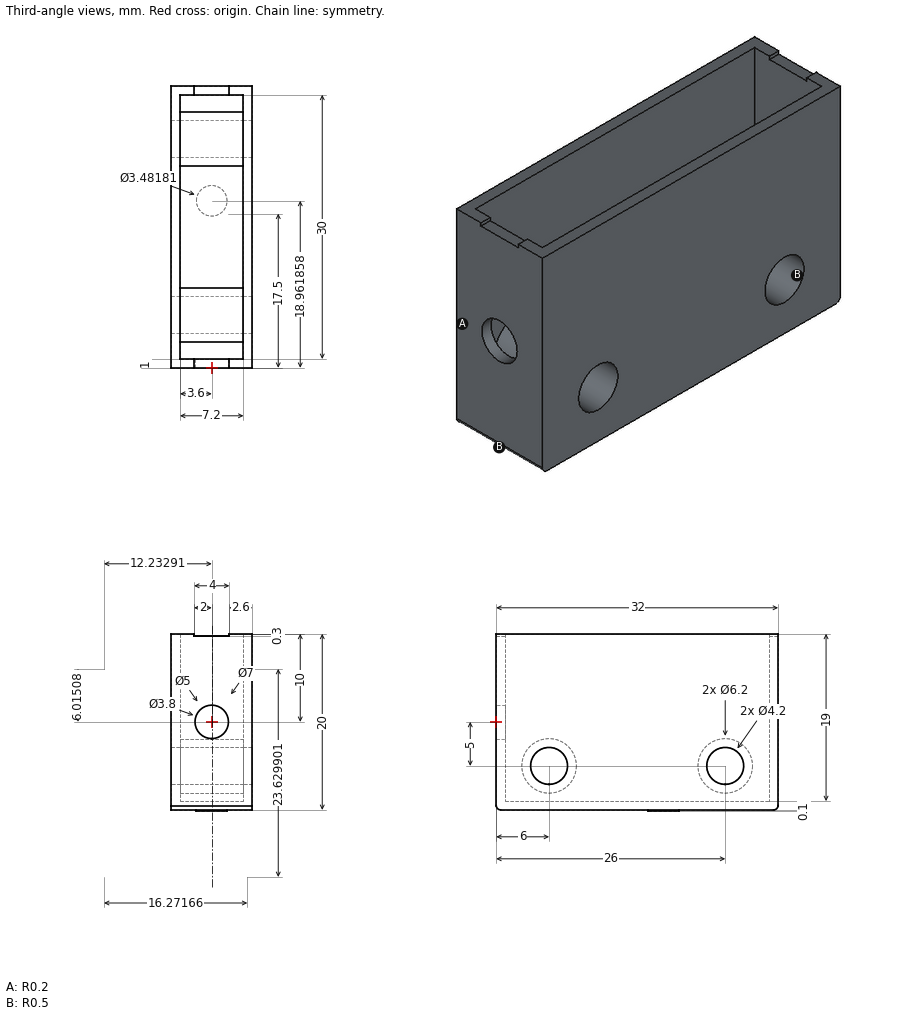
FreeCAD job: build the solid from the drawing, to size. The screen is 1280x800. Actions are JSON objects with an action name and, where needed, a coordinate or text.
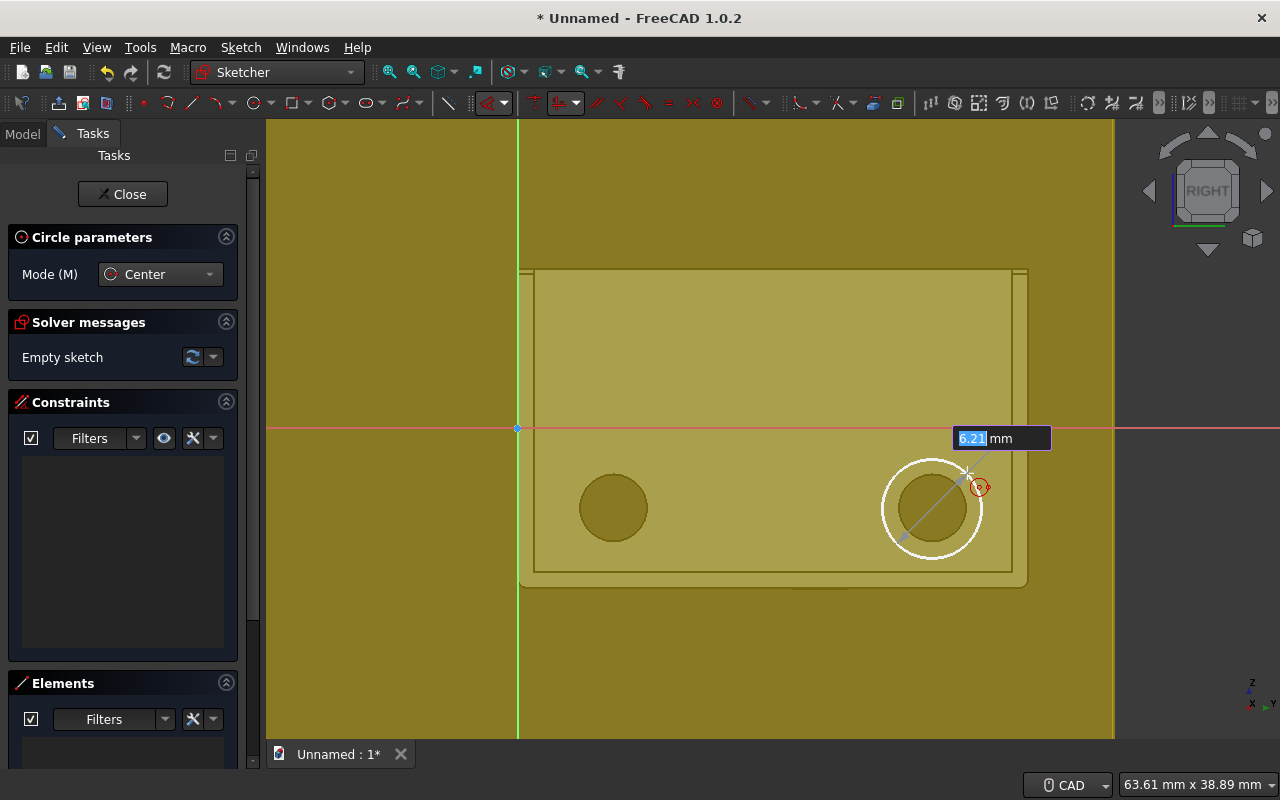
{"action": "type", "text": "6.2"}
{"action": "key", "text": "Return"}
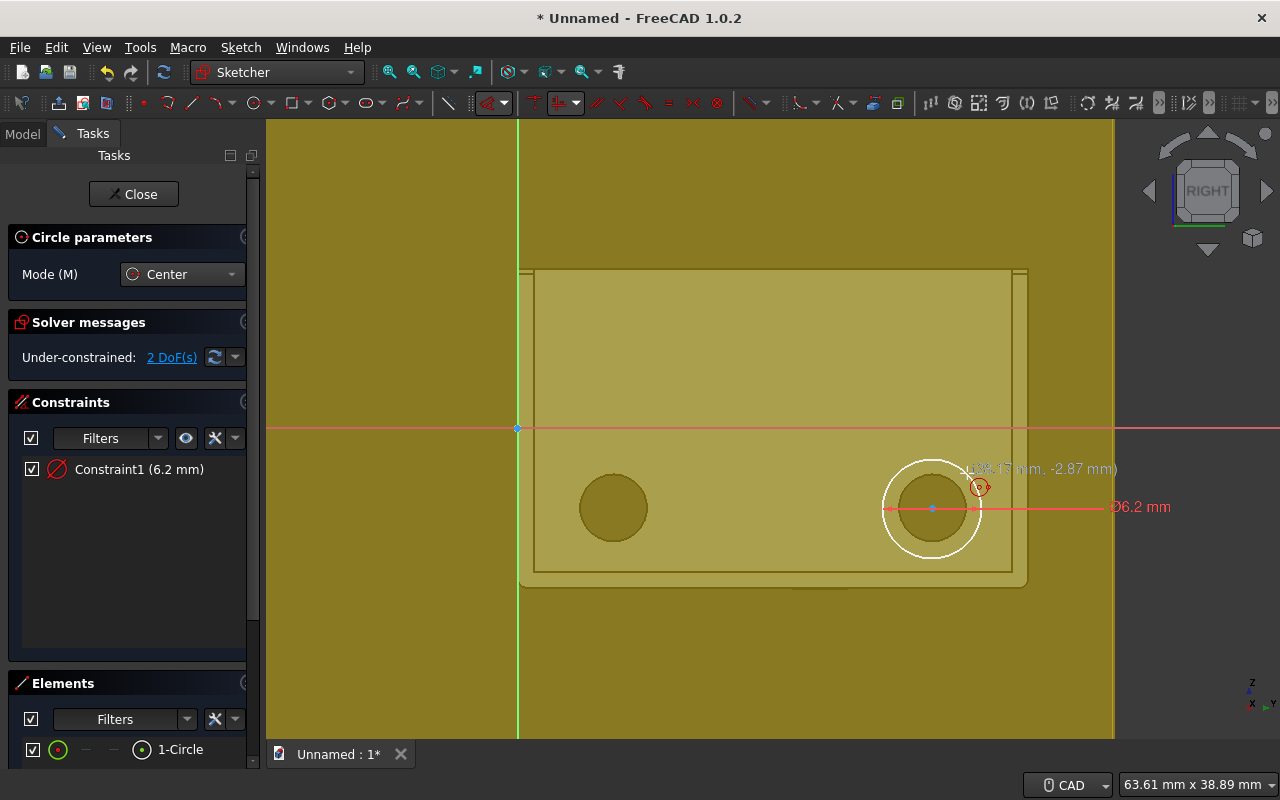
{"action": "left_click", "coordinate": [614, 508]}
{"action": "mouse_move", "coordinate": [649, 473]}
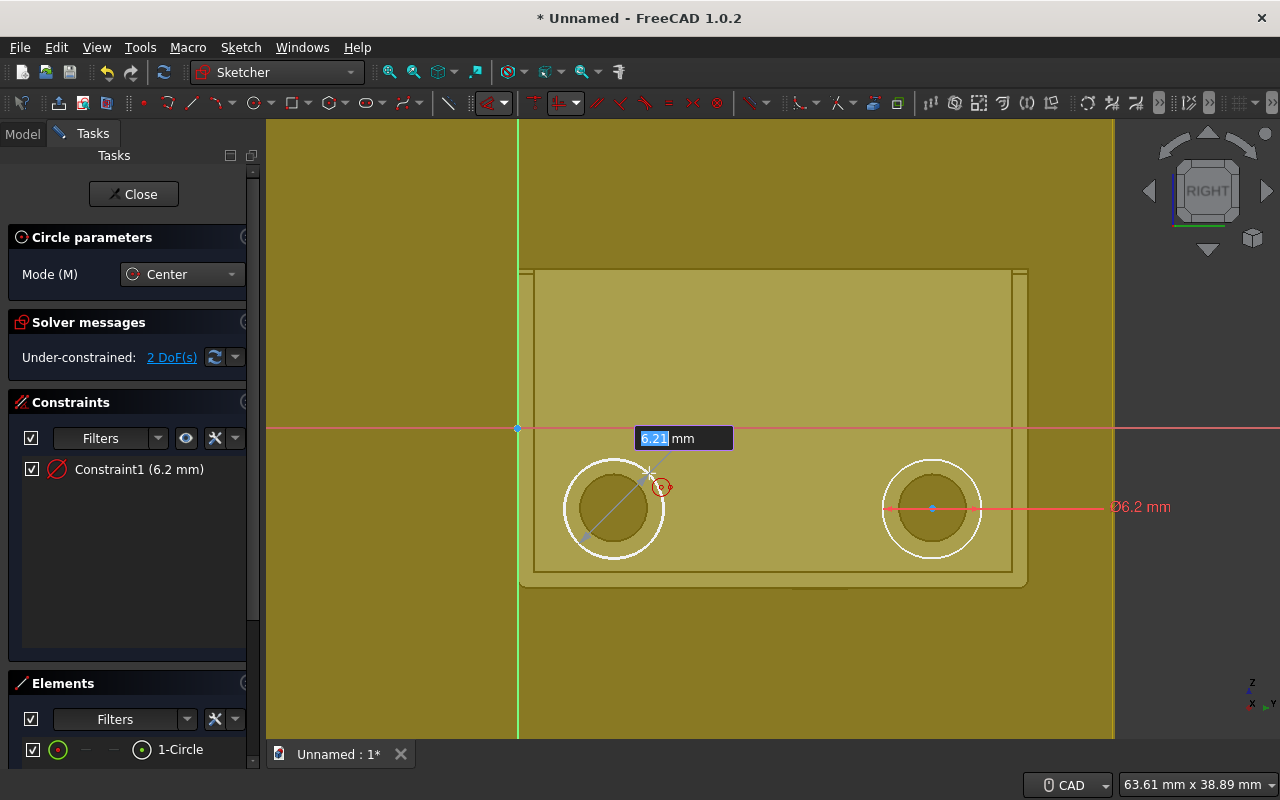
{"action": "type", "text": "6.2"}
{"action": "key", "text": "Return"}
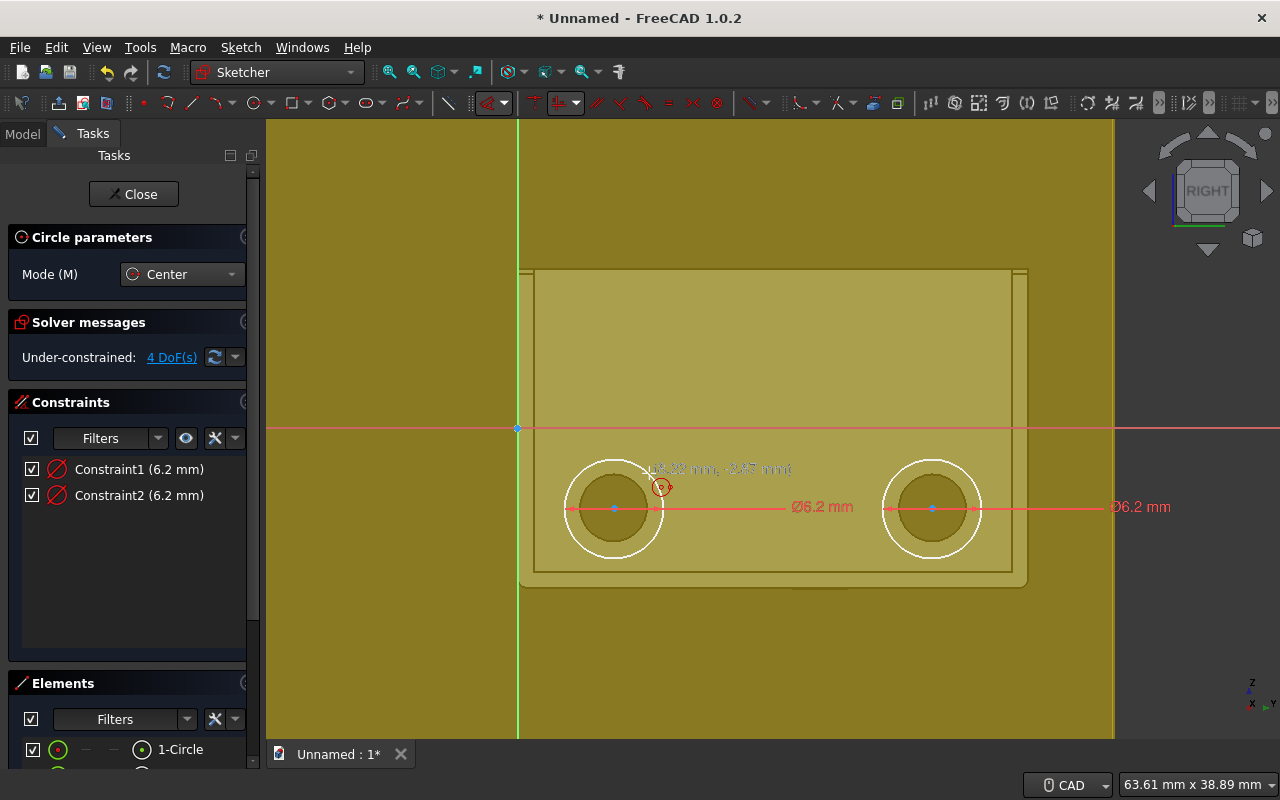
{"action": "left_click", "coordinate": [932, 509]}
{"action": "mouse_move", "coordinate": [956, 484]}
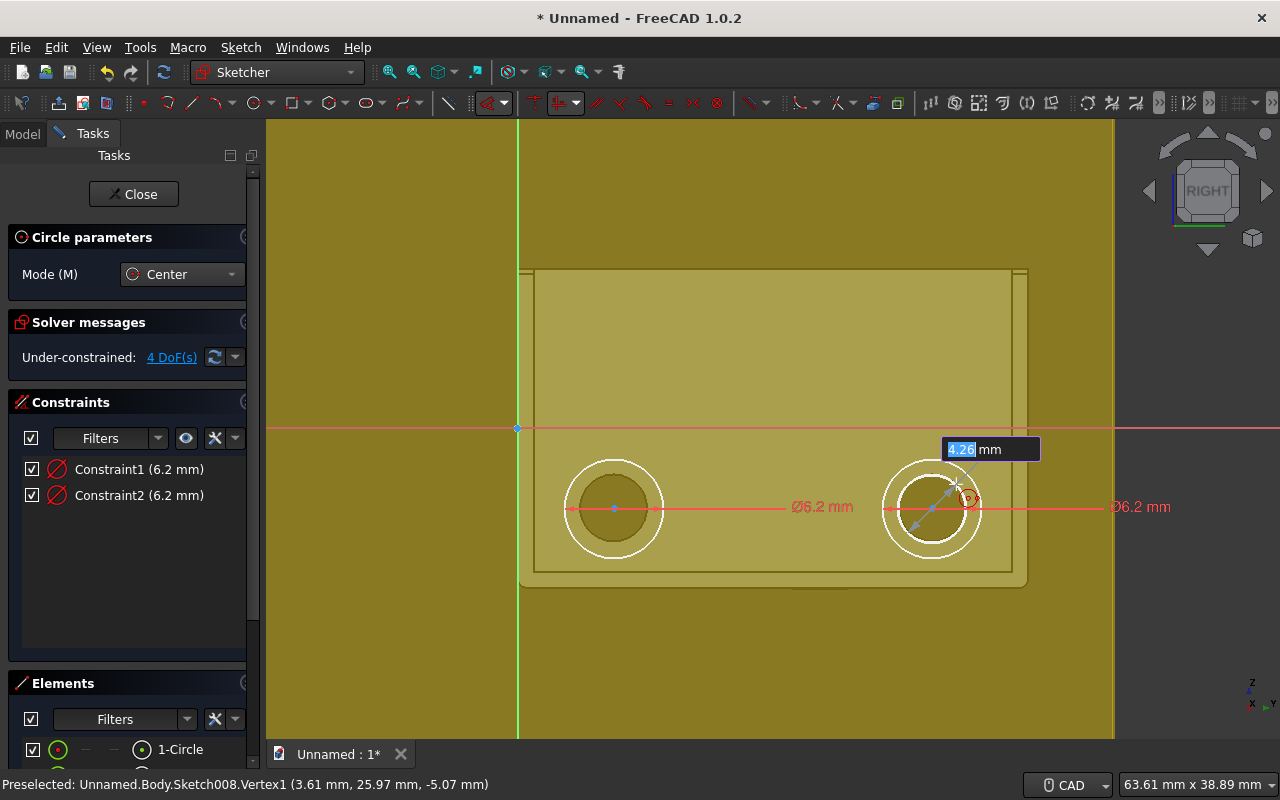
{"action": "type", "text": "4.2"}
{"action": "key", "text": "Return"}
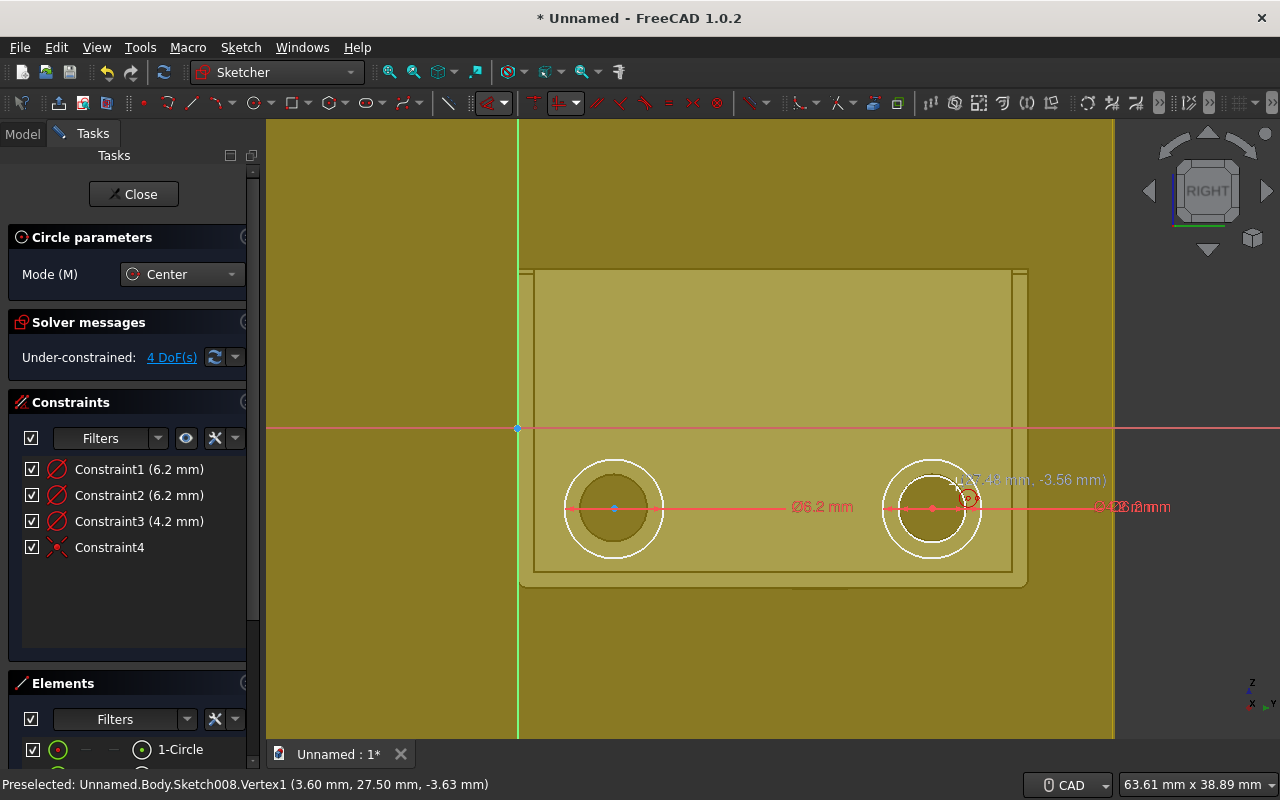
{"action": "left_click", "coordinate": [614, 509]}
{"action": "mouse_move", "coordinate": [637, 484]}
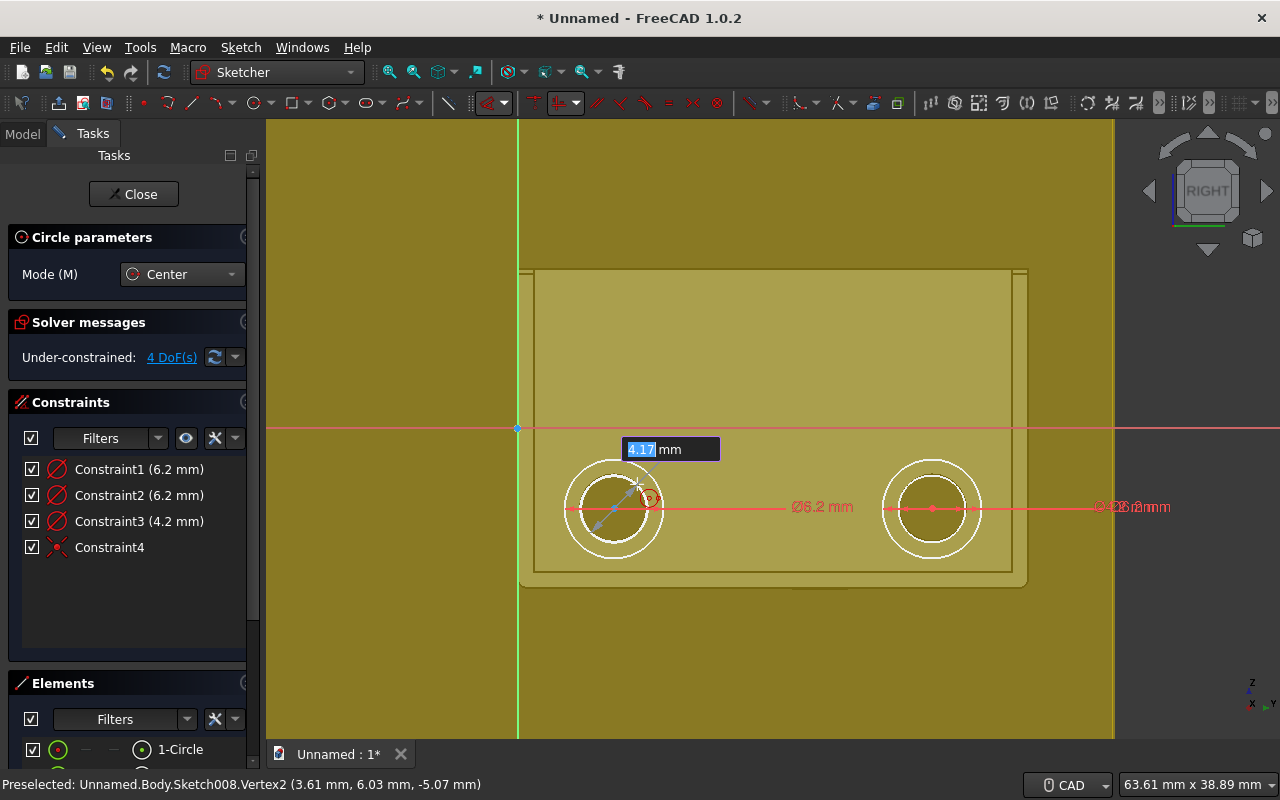
{"action": "type", "text": "4.2"}
{"action": "key", "text": "Return"}
{"action": "key", "text": "Escape"}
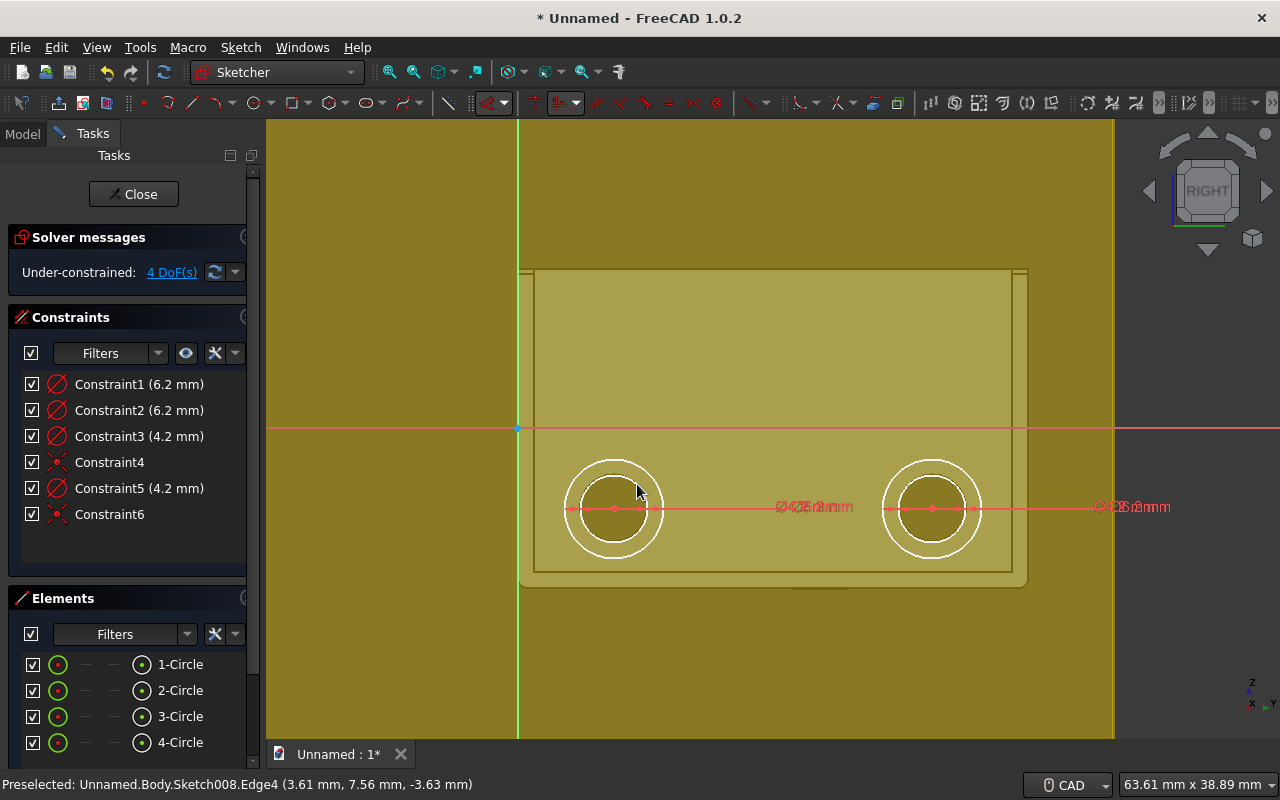
{"action": "left_click", "coordinate": [932, 509]}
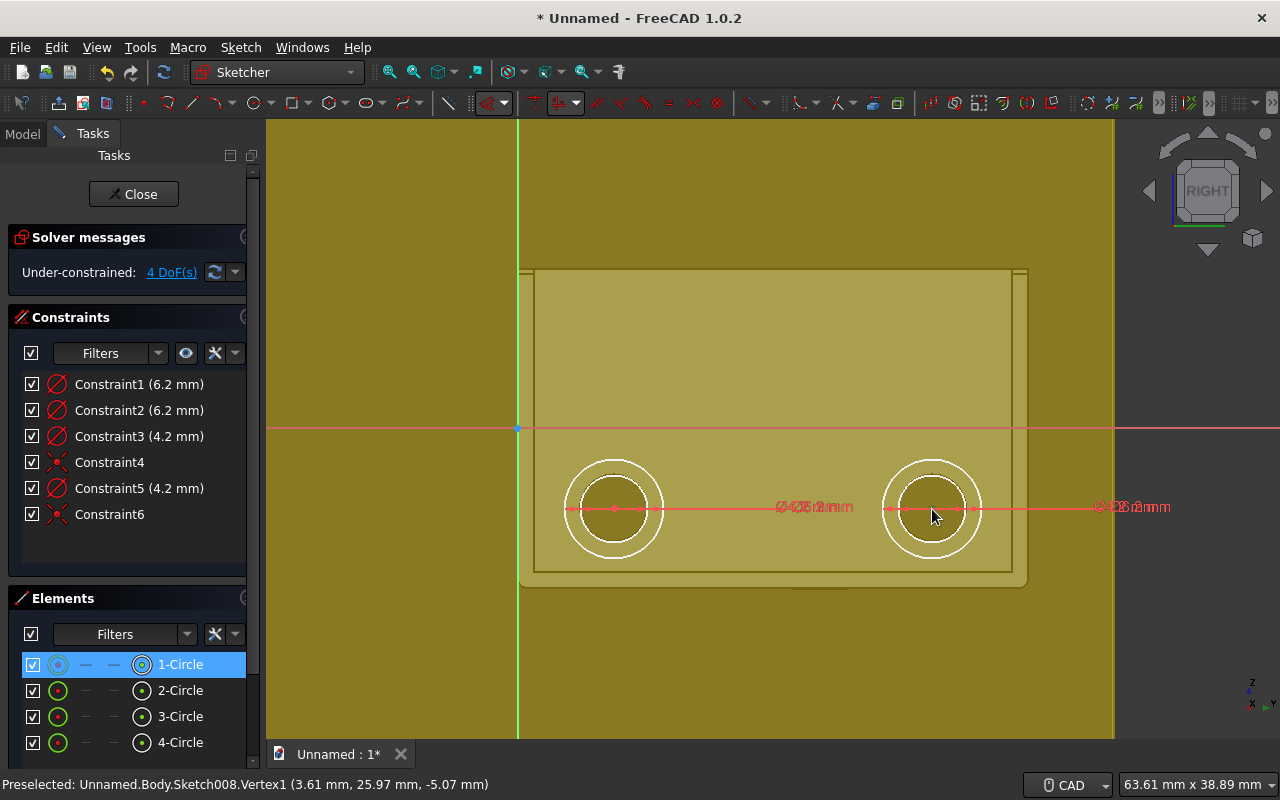
{"action": "left_click", "coordinate": [614, 509]}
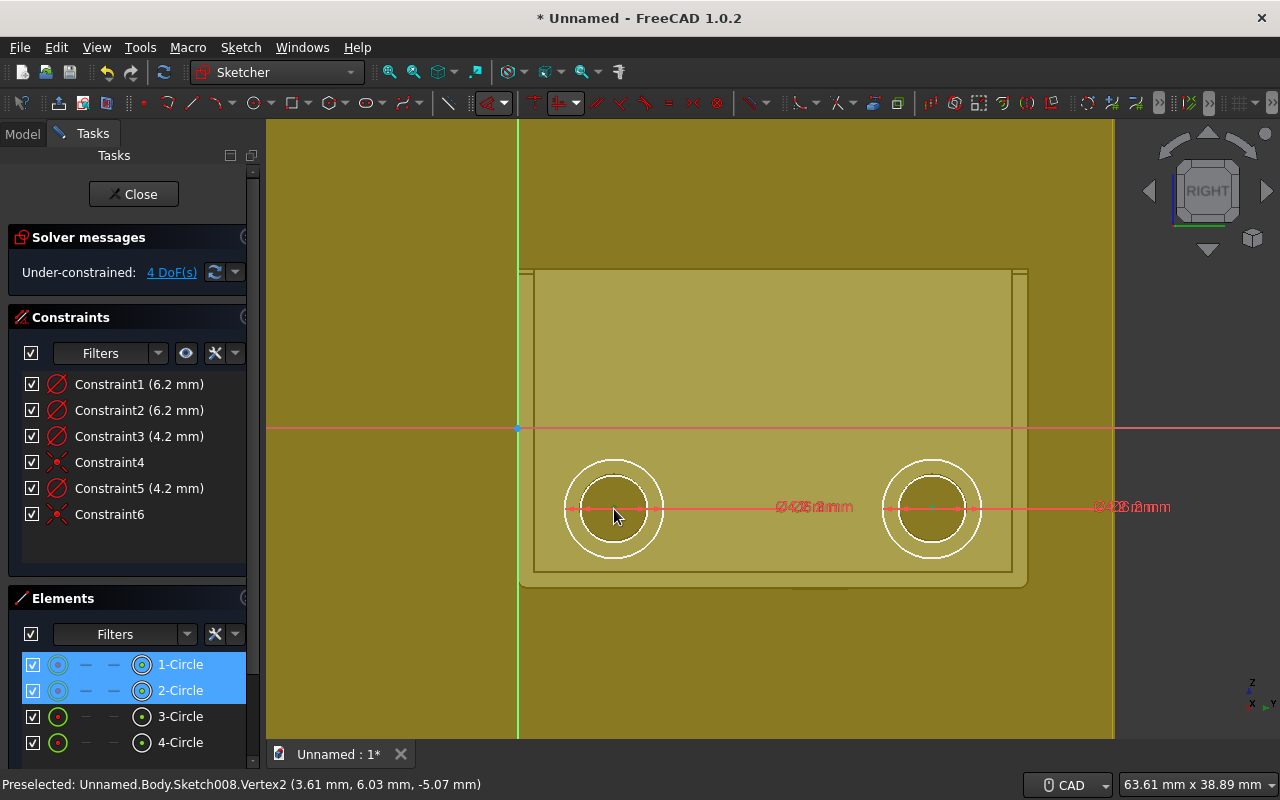
{"action": "left_click", "coordinate": [578, 104]}